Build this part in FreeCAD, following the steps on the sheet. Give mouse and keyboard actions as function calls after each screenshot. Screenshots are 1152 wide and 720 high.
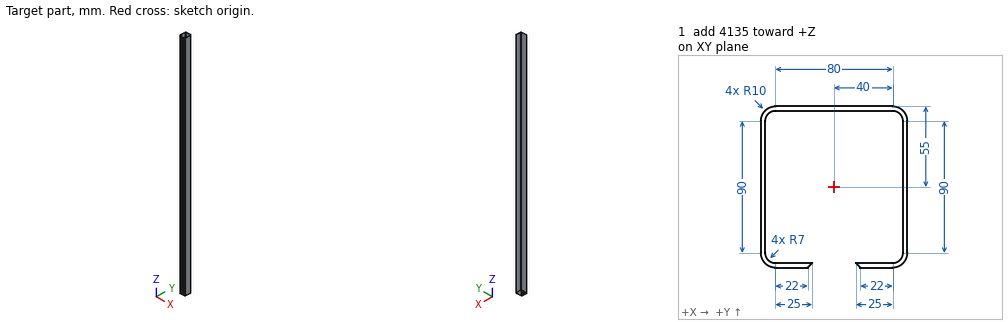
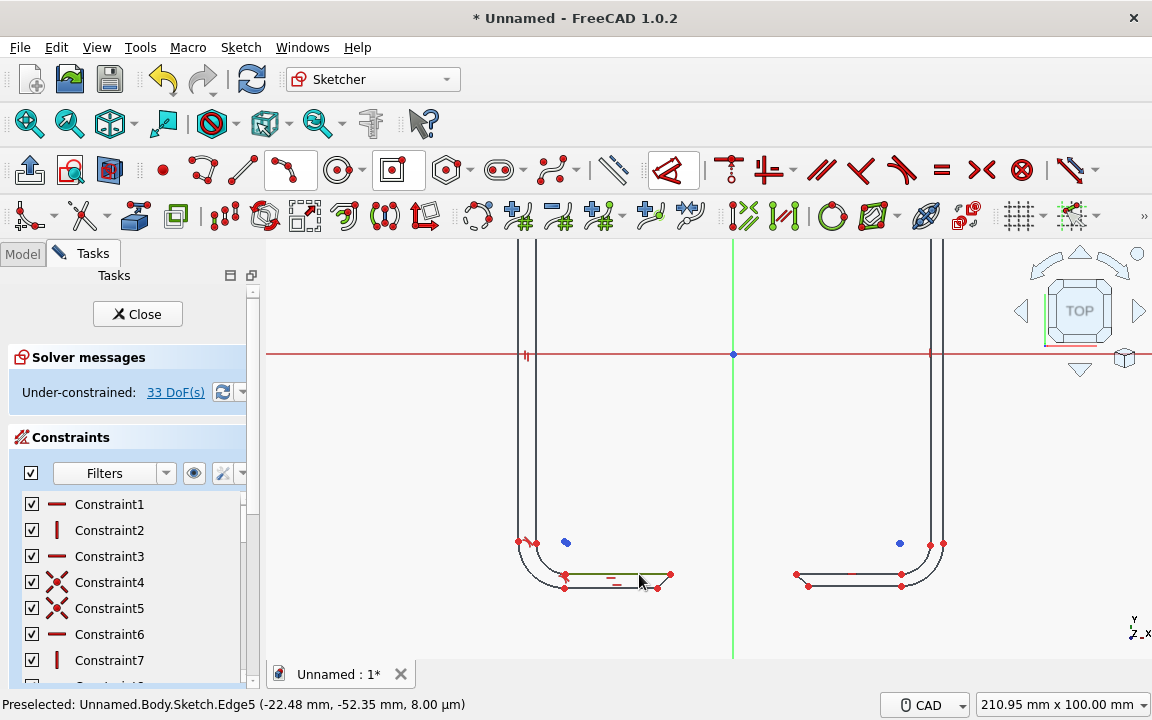
click(540, 557)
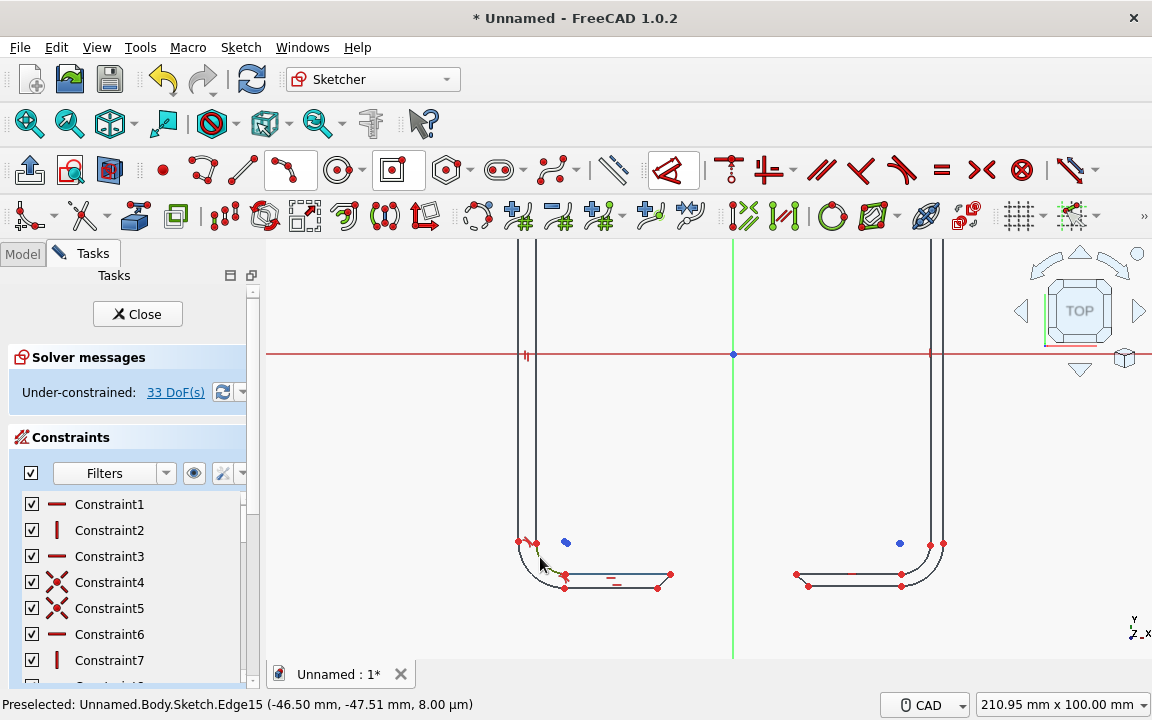
click(902, 170)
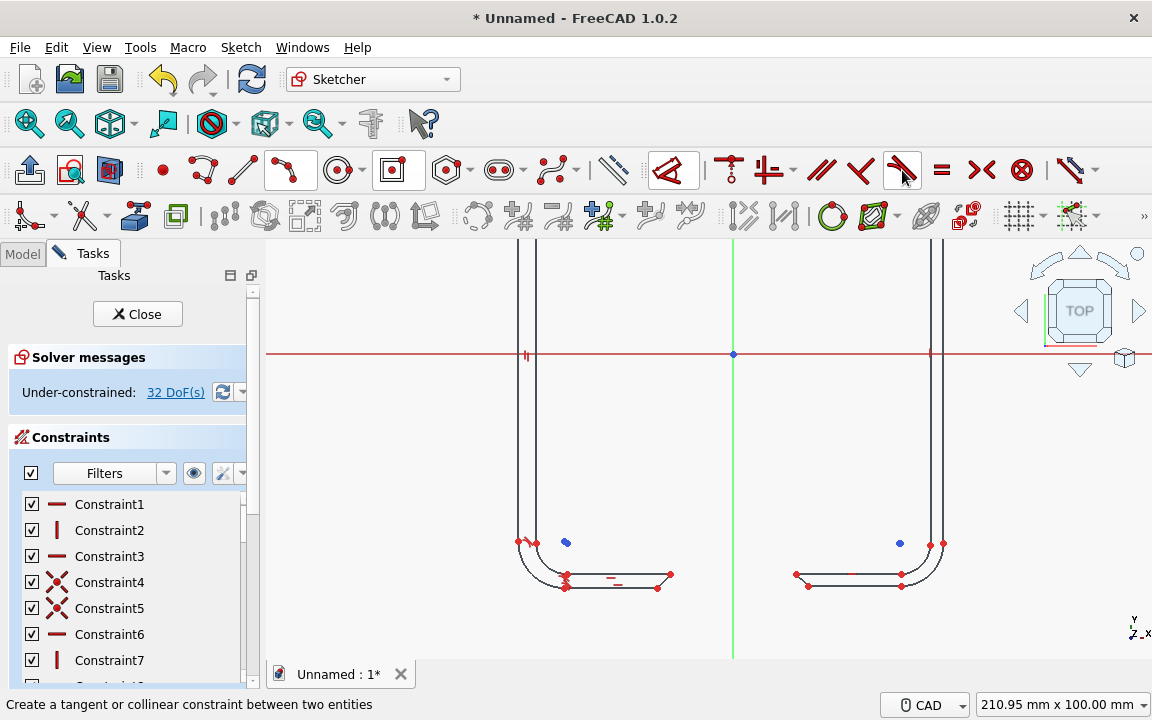
click(536, 431)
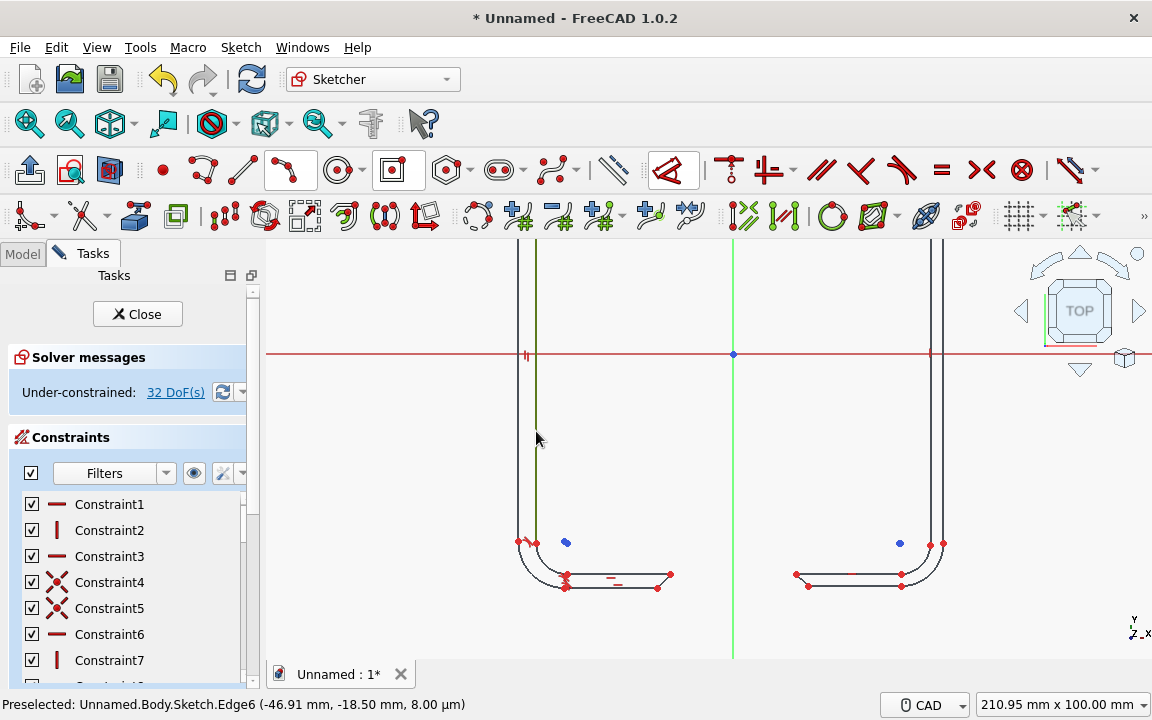
click(540, 558)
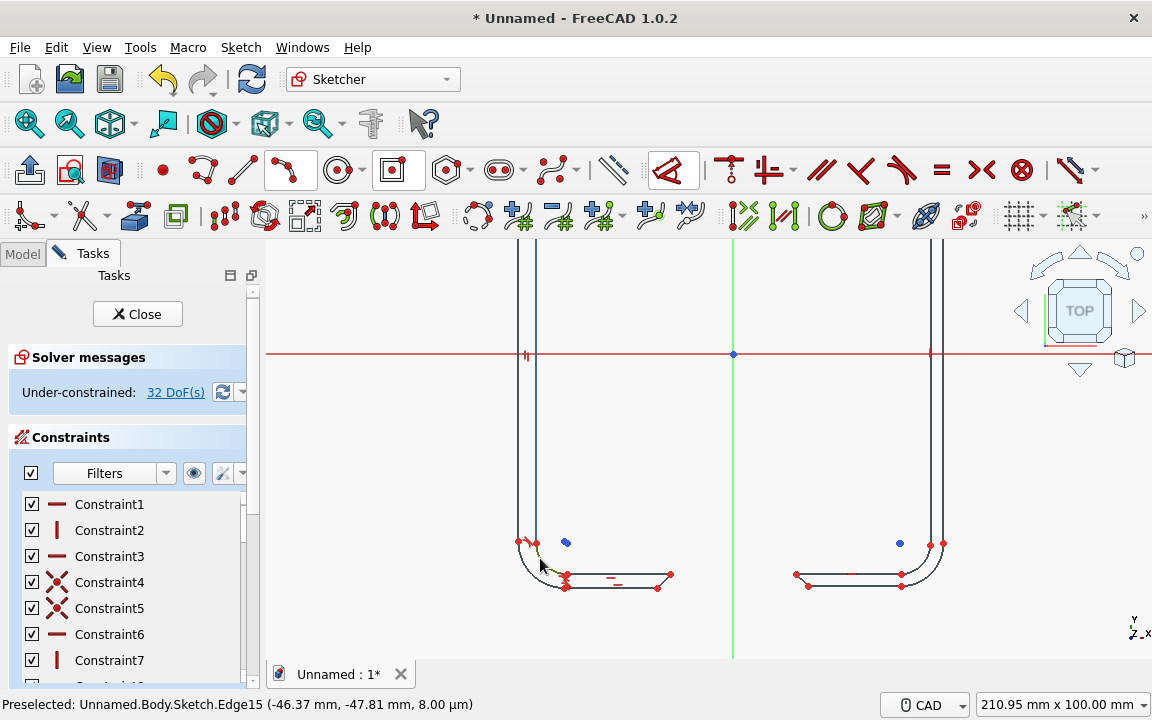
click(902, 170)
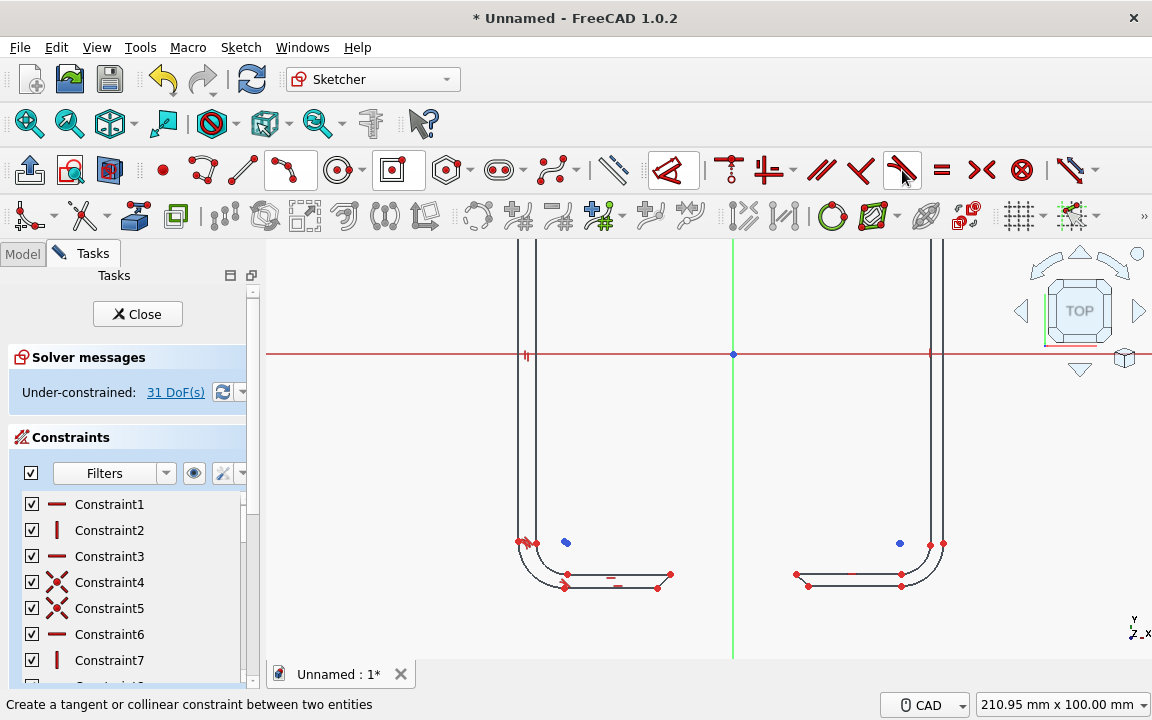
click(536, 431)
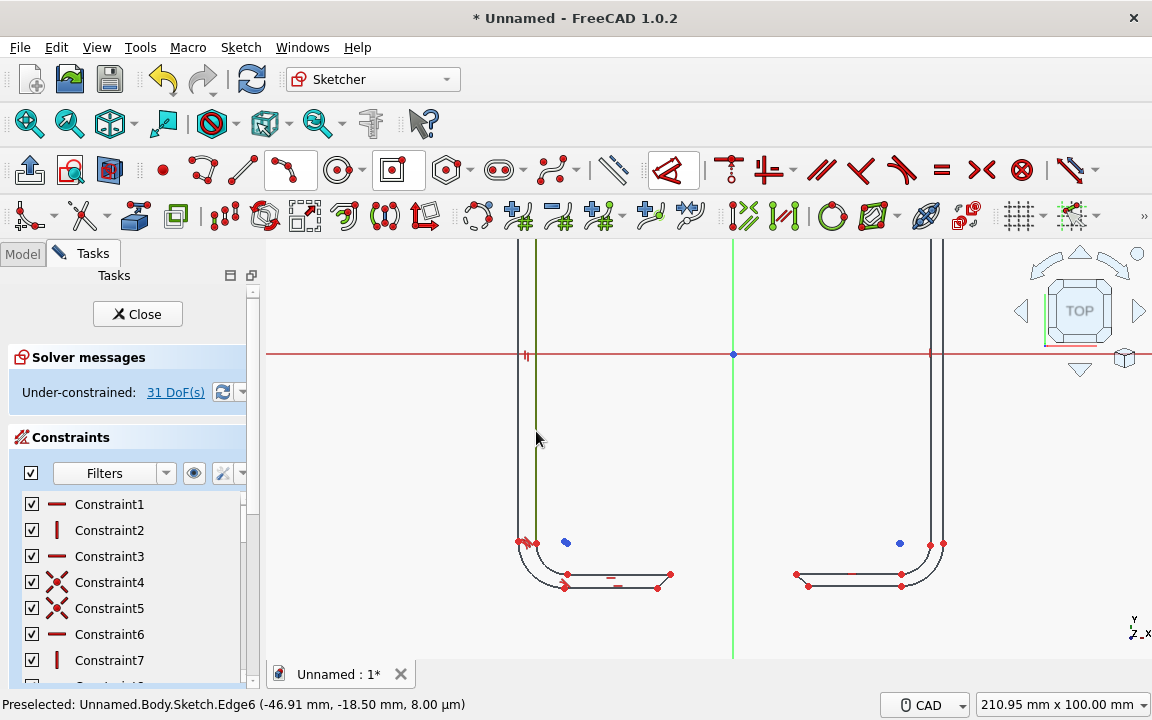
scroll(527, 564, down, 3)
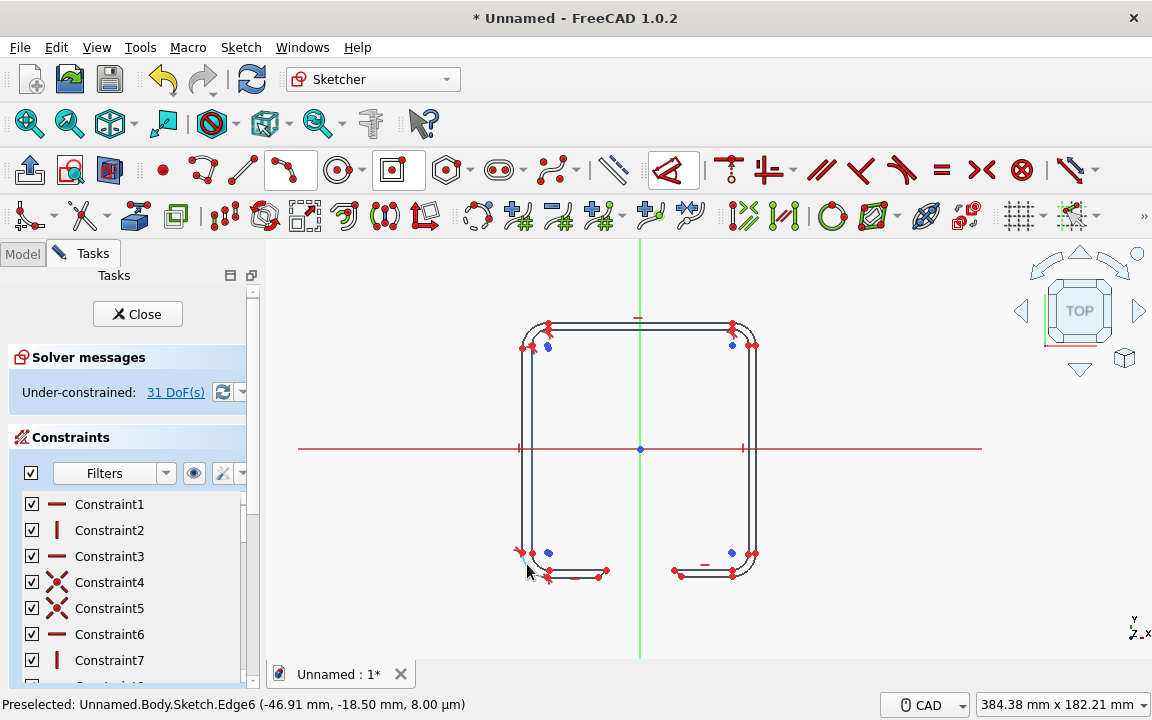
scroll(541, 331, up, 4)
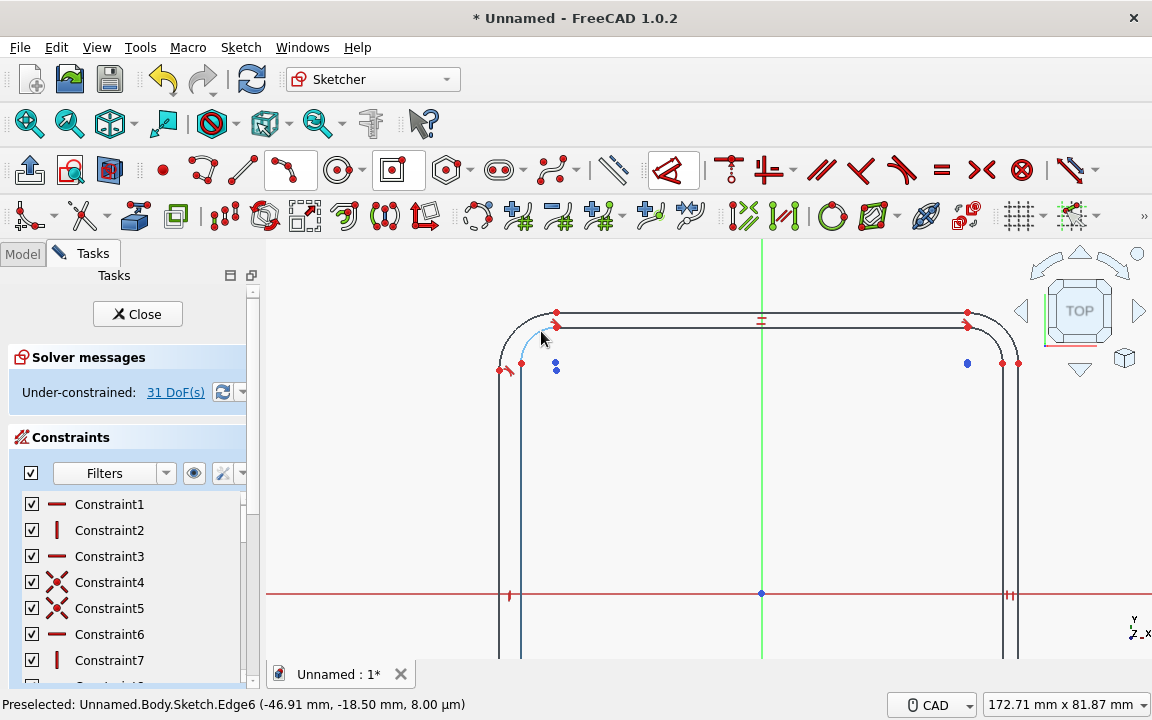
click(540, 331)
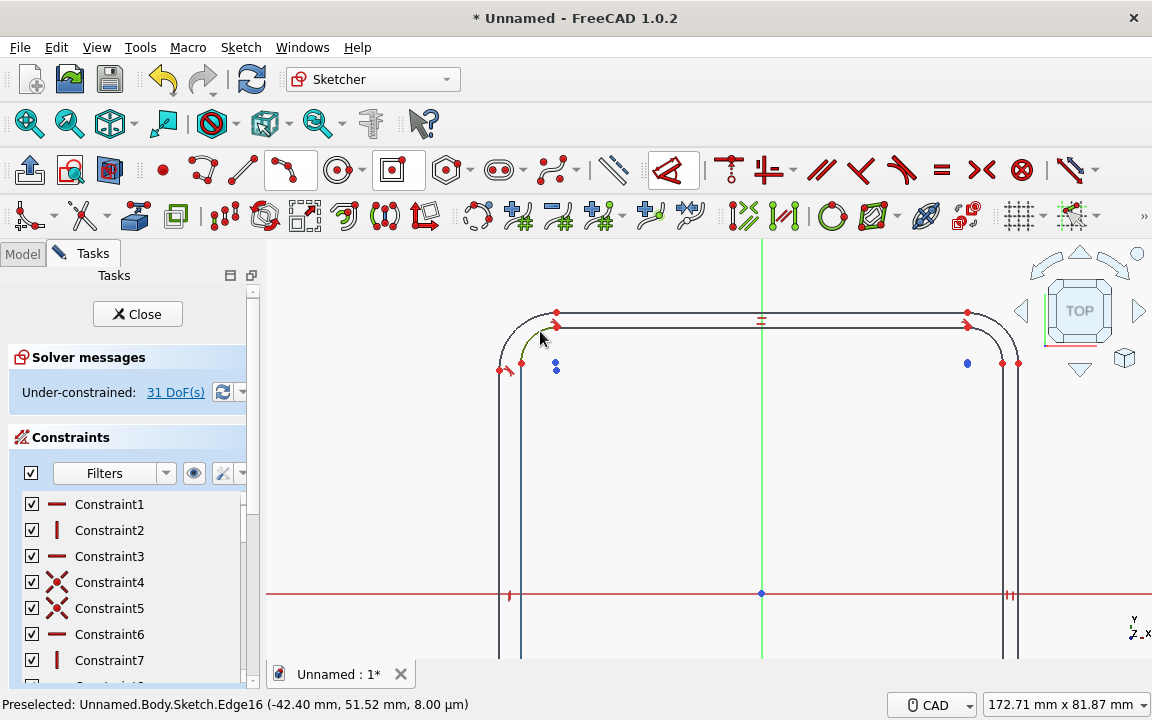
click(902, 170)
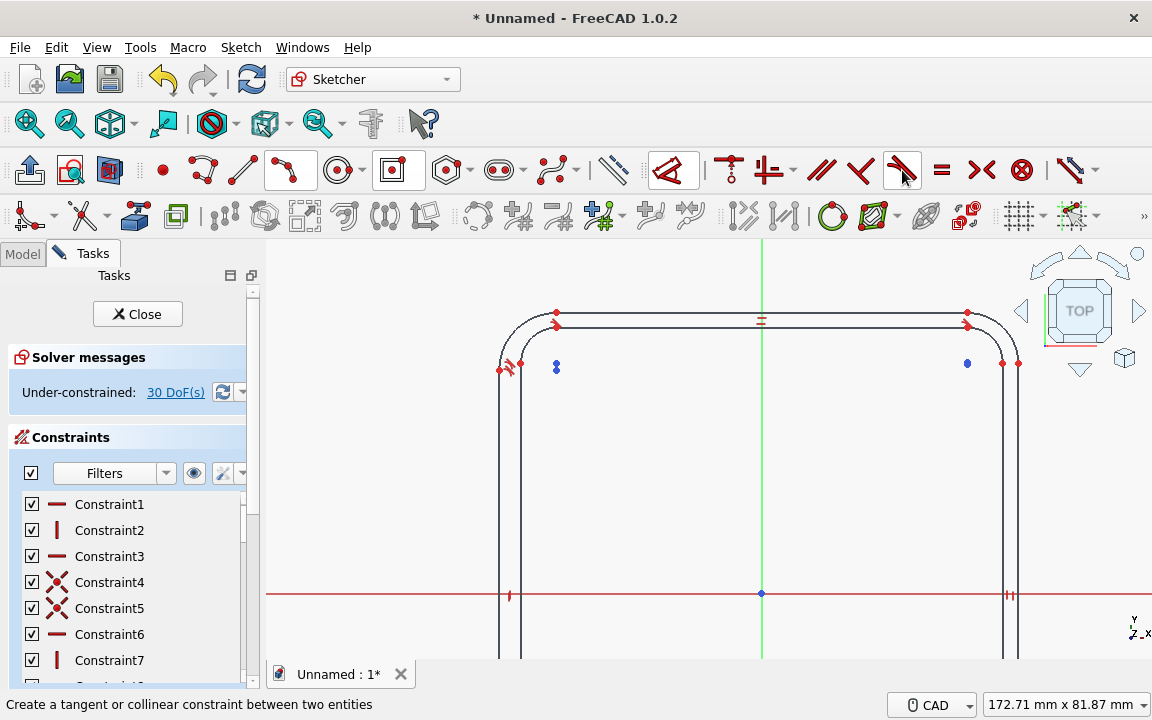
click(680, 328)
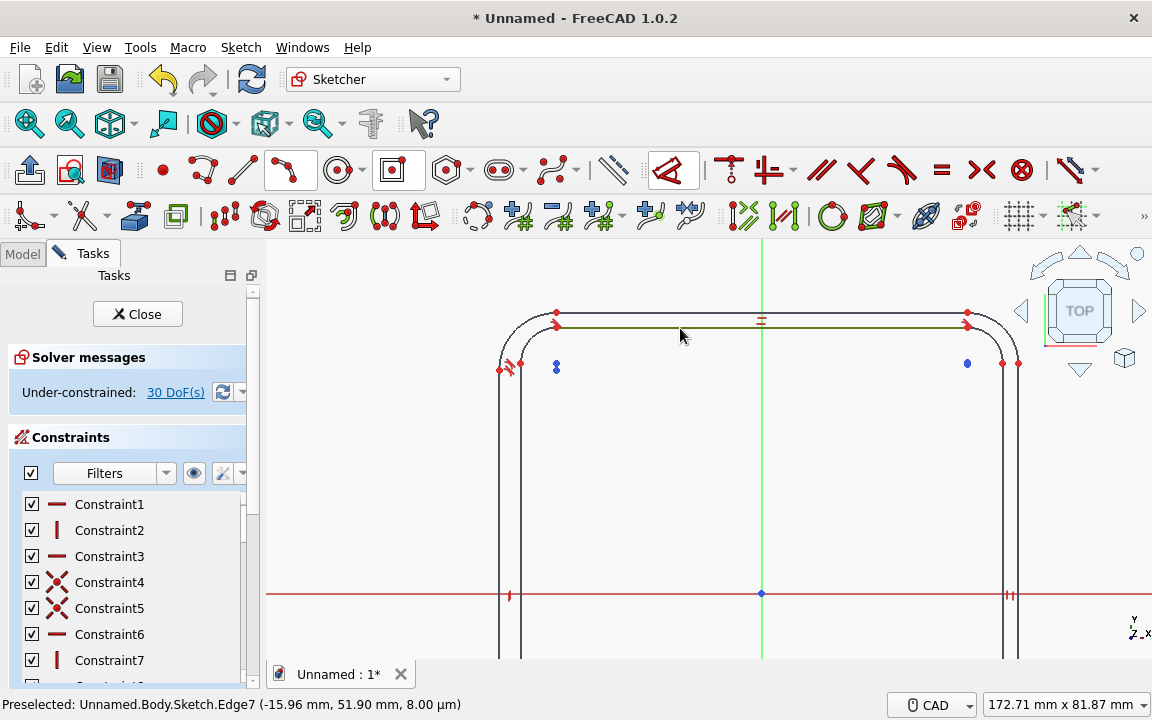
click(540, 332)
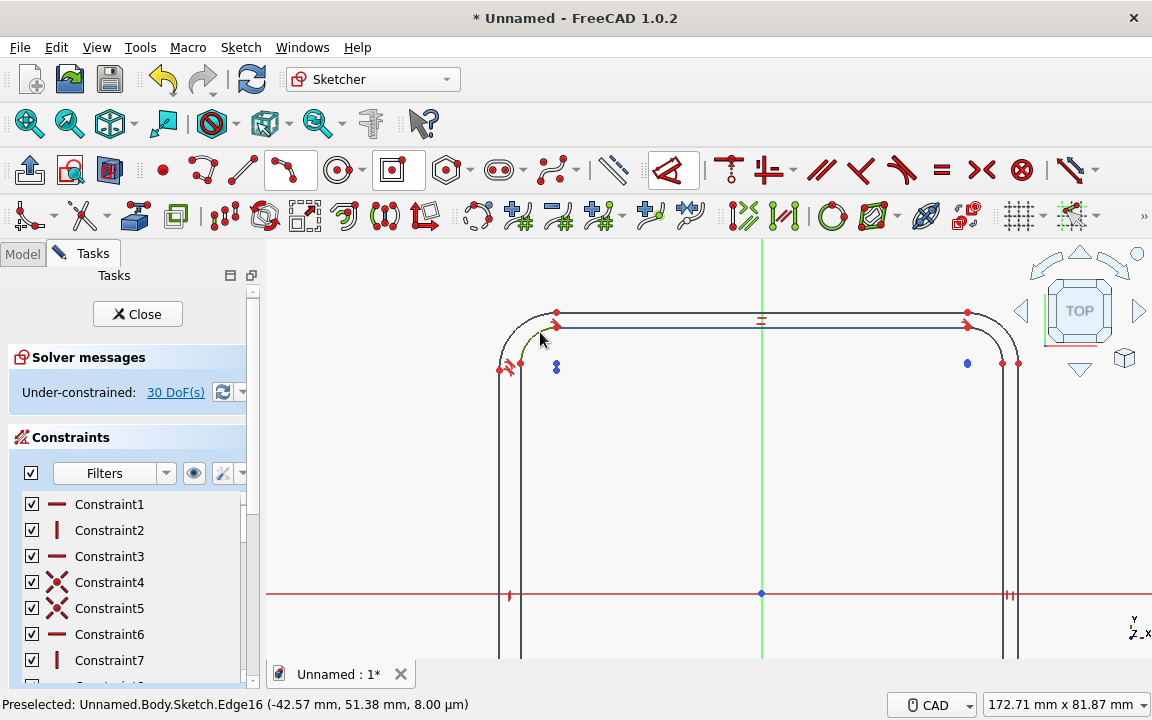
click(902, 170)